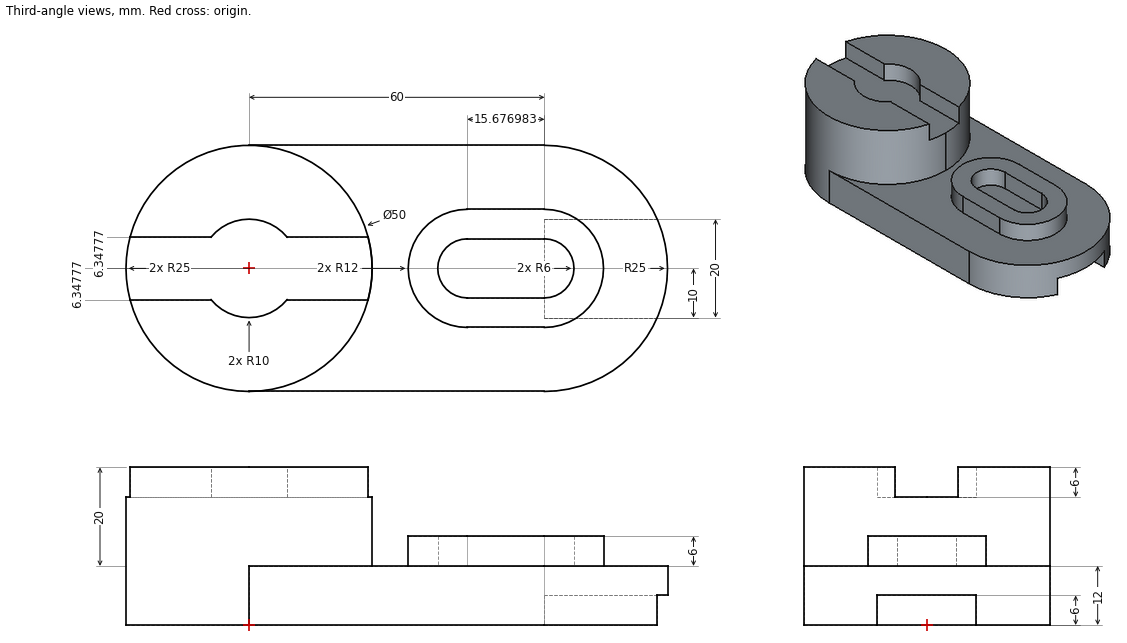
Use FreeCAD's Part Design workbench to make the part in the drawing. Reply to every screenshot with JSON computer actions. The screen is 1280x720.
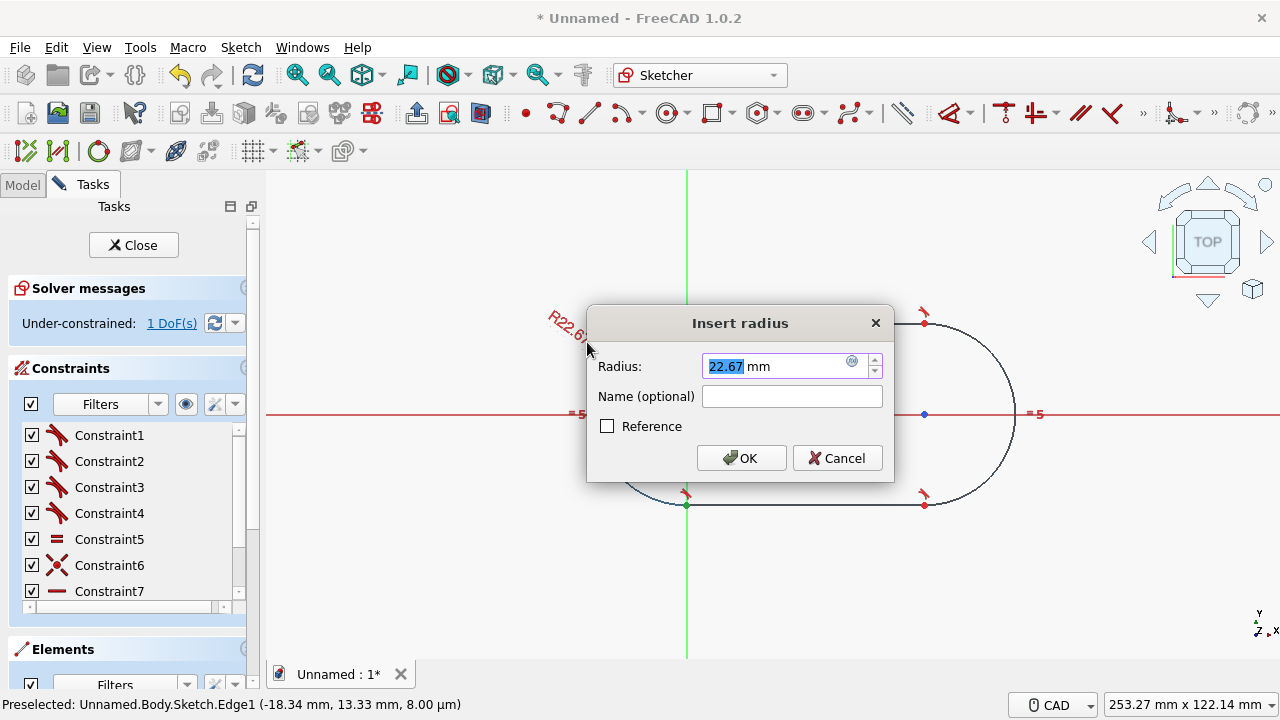
{"action": "type", "text": "25"}
{"action": "key", "text": "Return"}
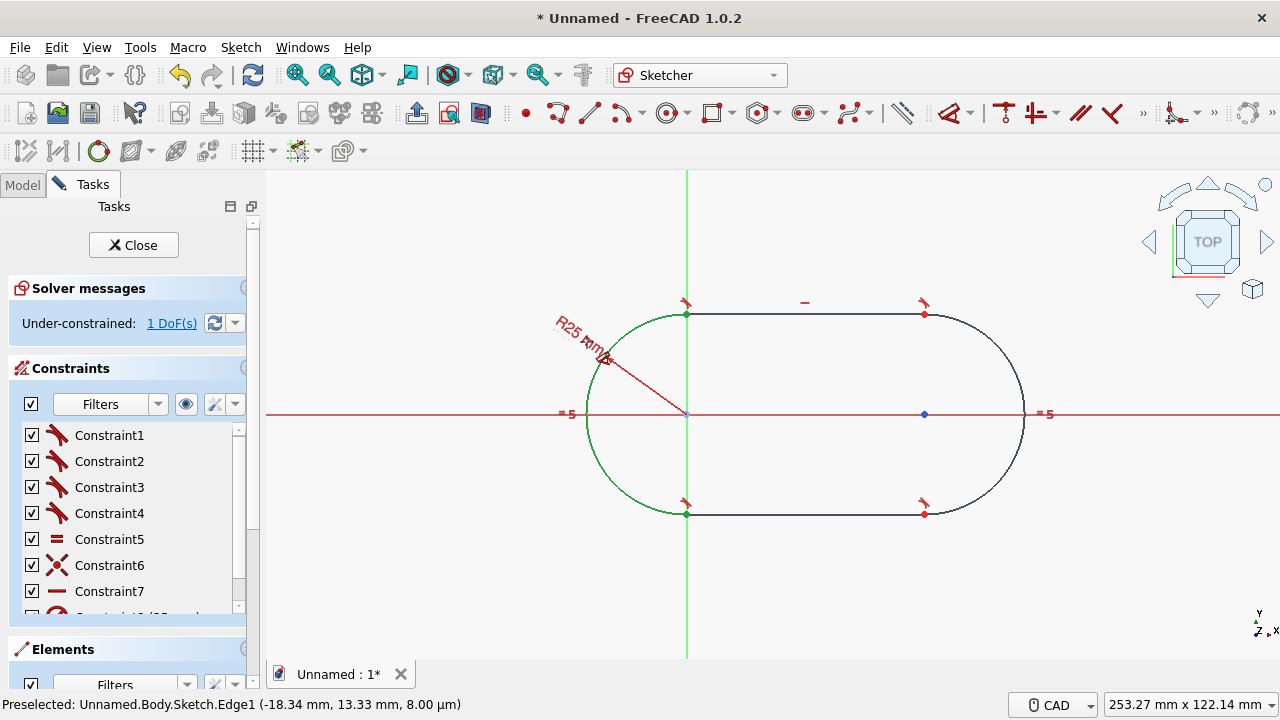
{"action": "left_click", "coordinate": [758, 314]}
{"action": "left_click", "coordinate": [806, 280]}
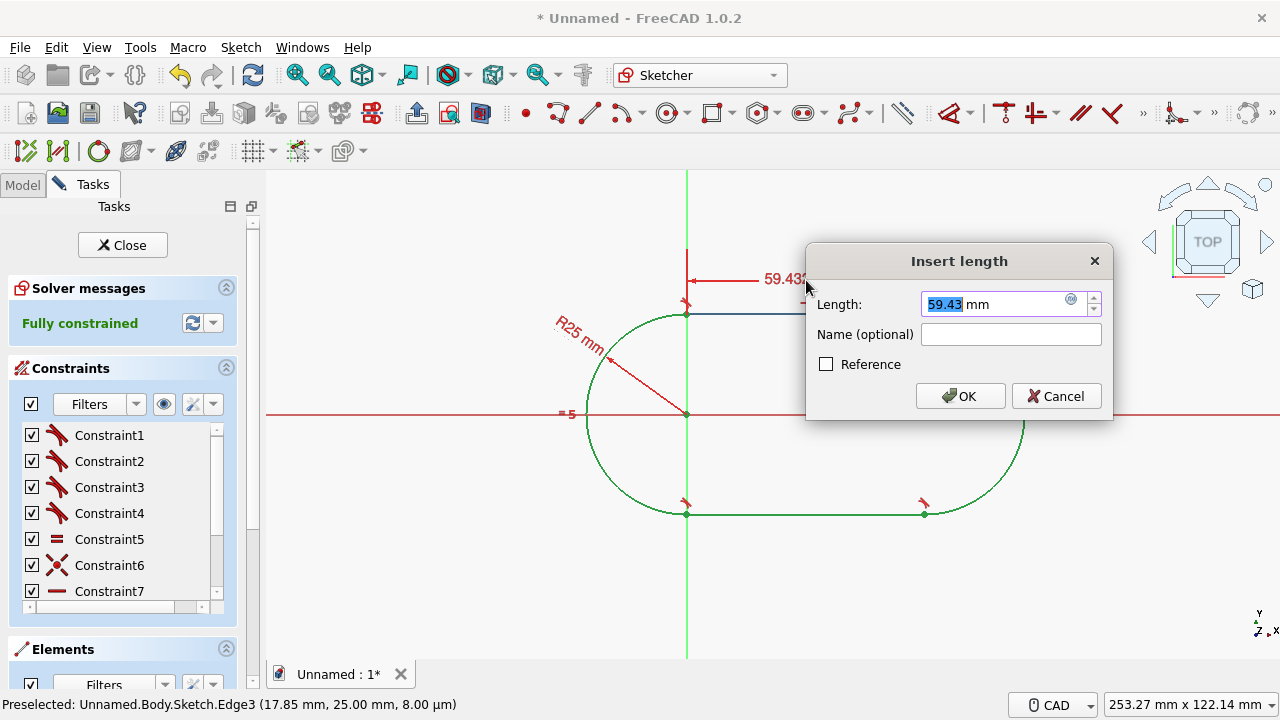
{"action": "type", "text": "60"}
{"action": "key", "text": "Return"}
{"action": "key", "text": "Escape"}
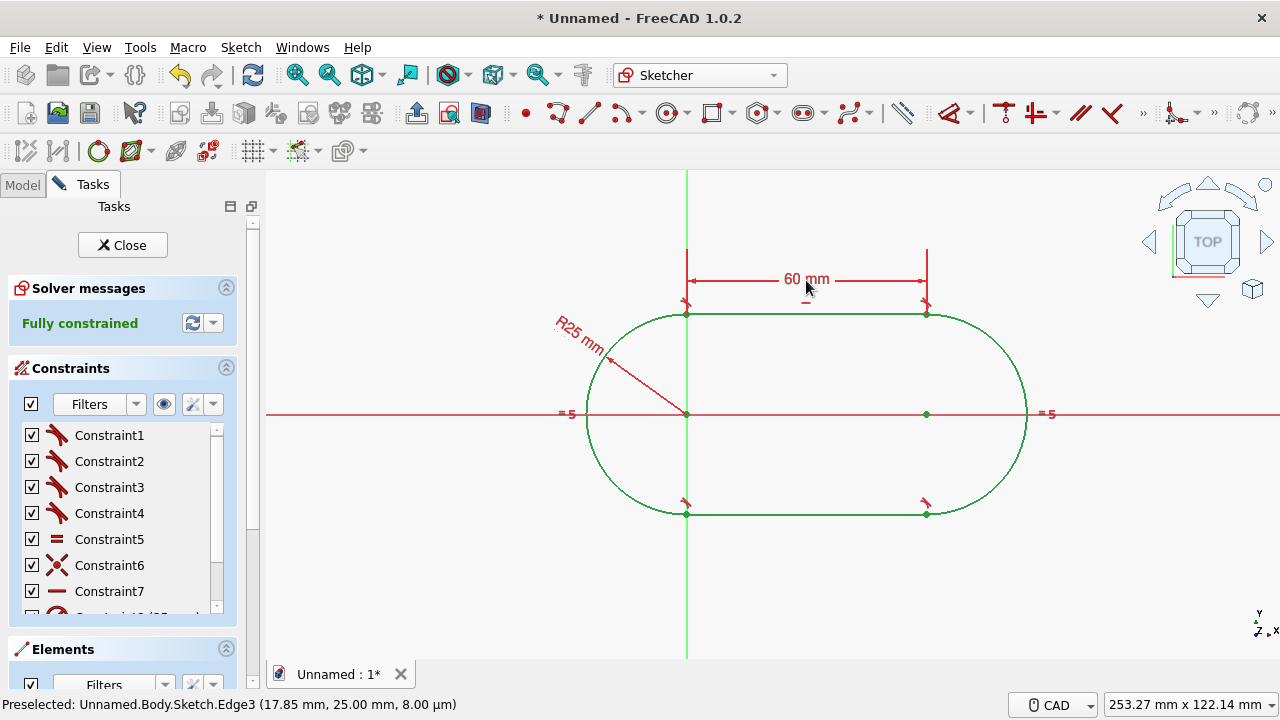
{"action": "left_click", "coordinate": [123, 245]}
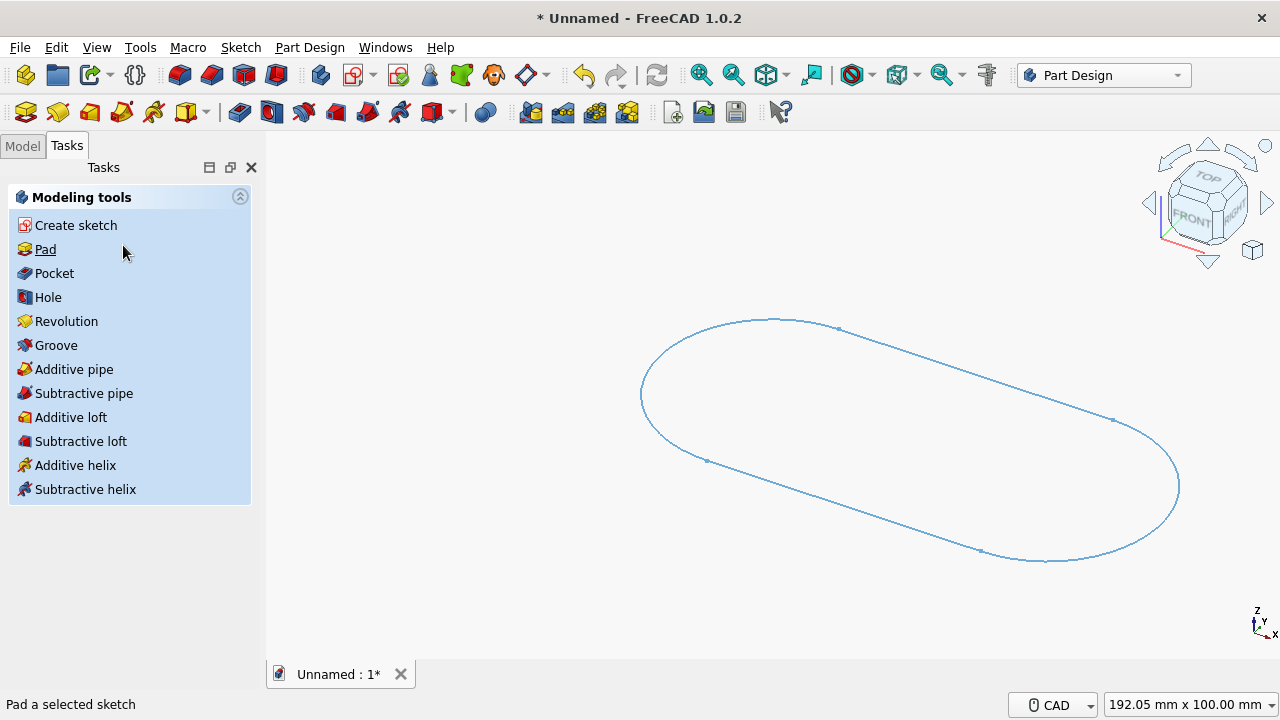
{"action": "left_click", "coordinate": [26, 112]}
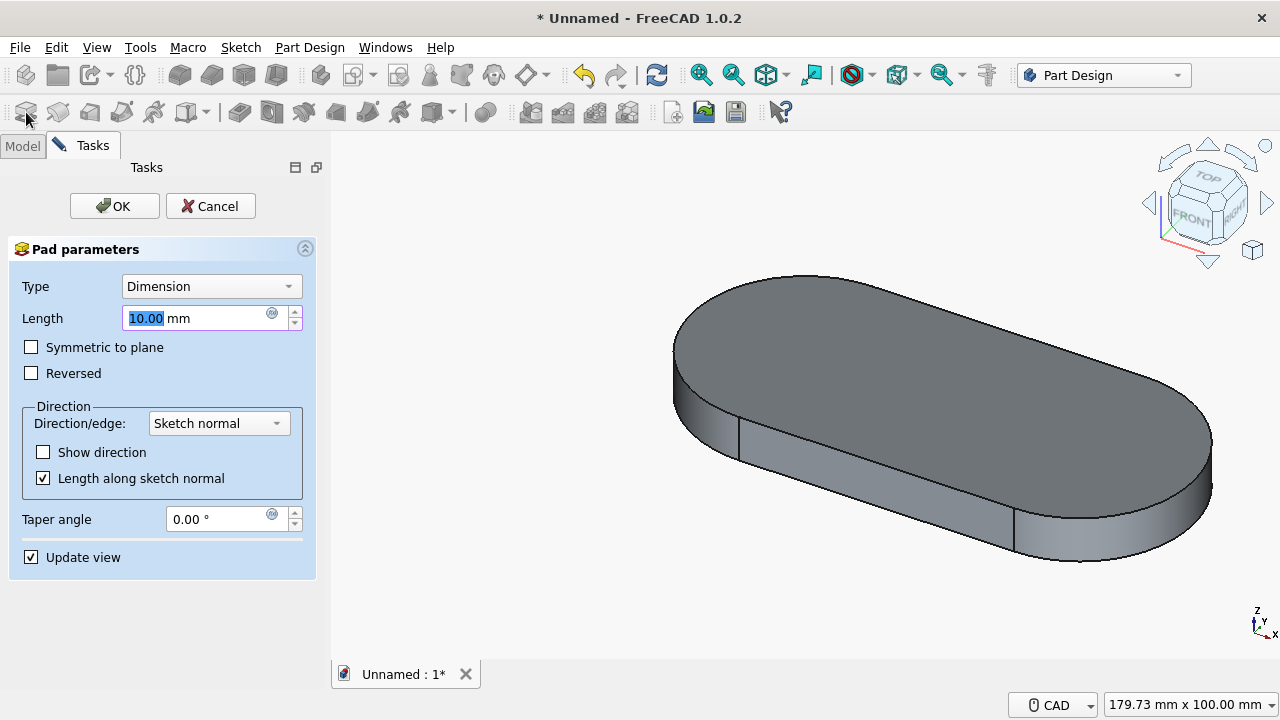
{"action": "type", "text": "12"}
{"action": "key", "text": "Tab"}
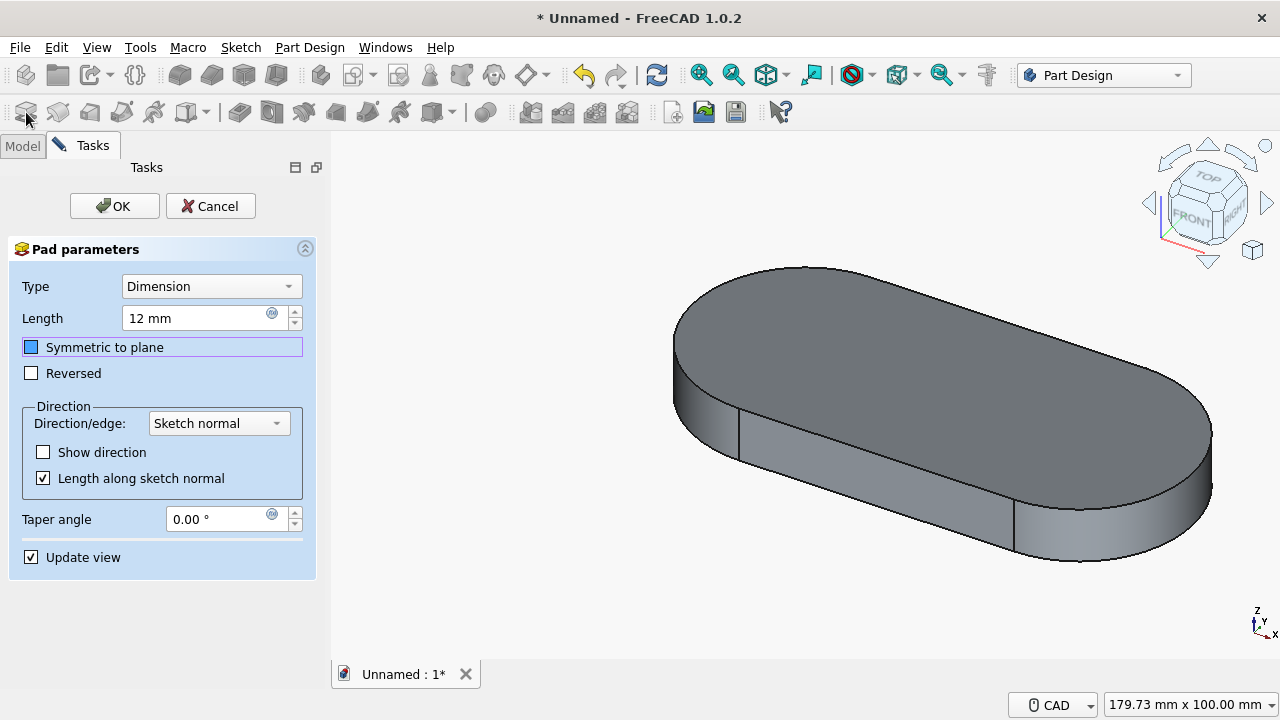
{"action": "left_click", "coordinate": [115, 206]}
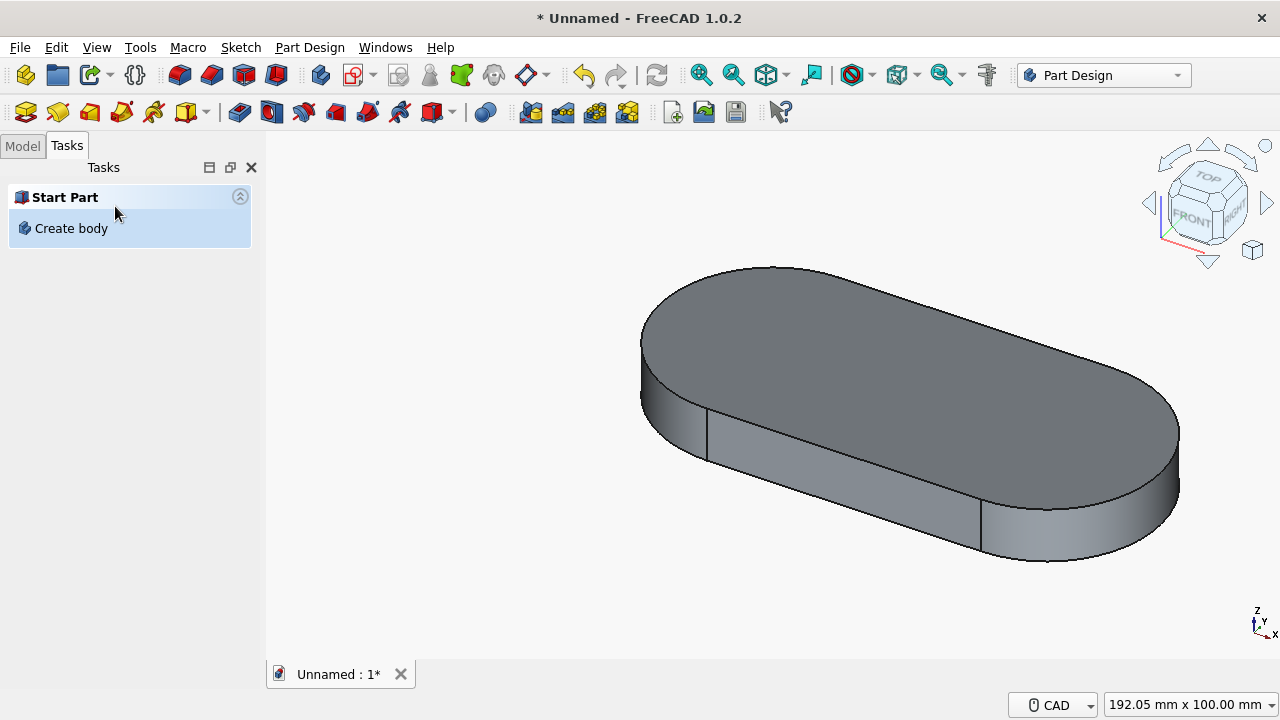
{"action": "left_click", "coordinate": [982, 411]}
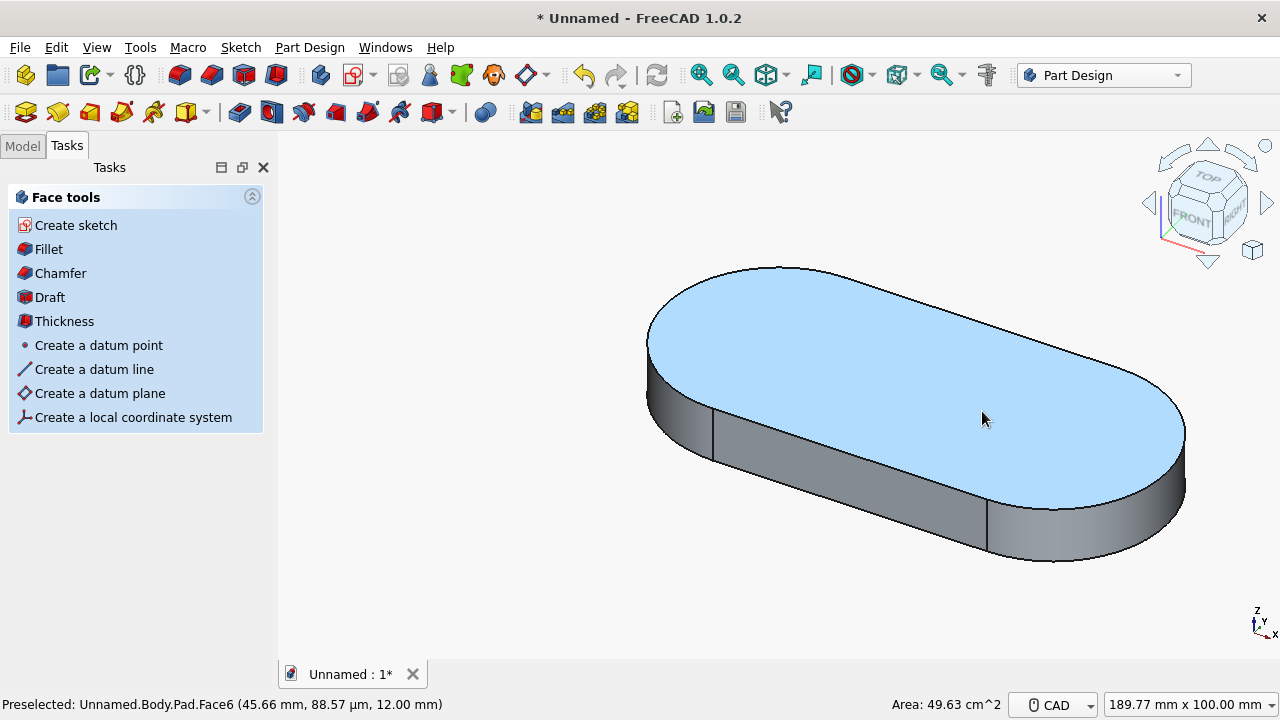
{"action": "left_click", "coordinate": [354, 76]}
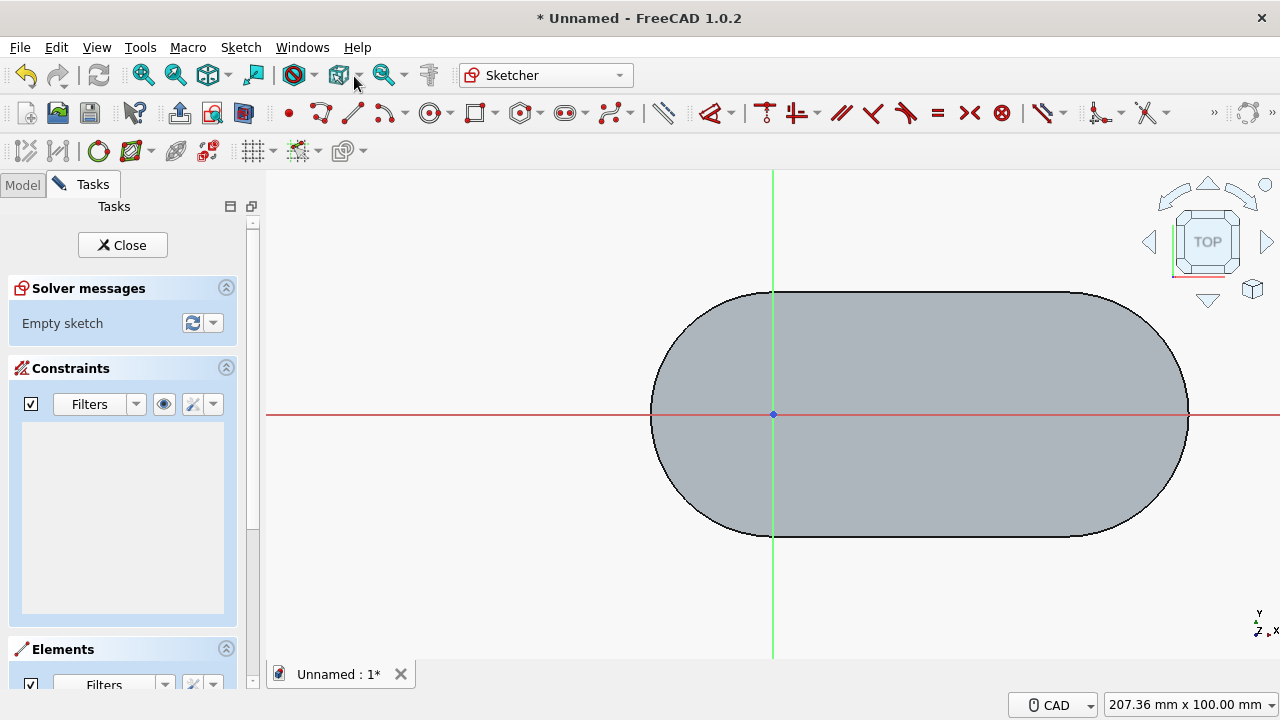
{"action": "key", "text": "g c"}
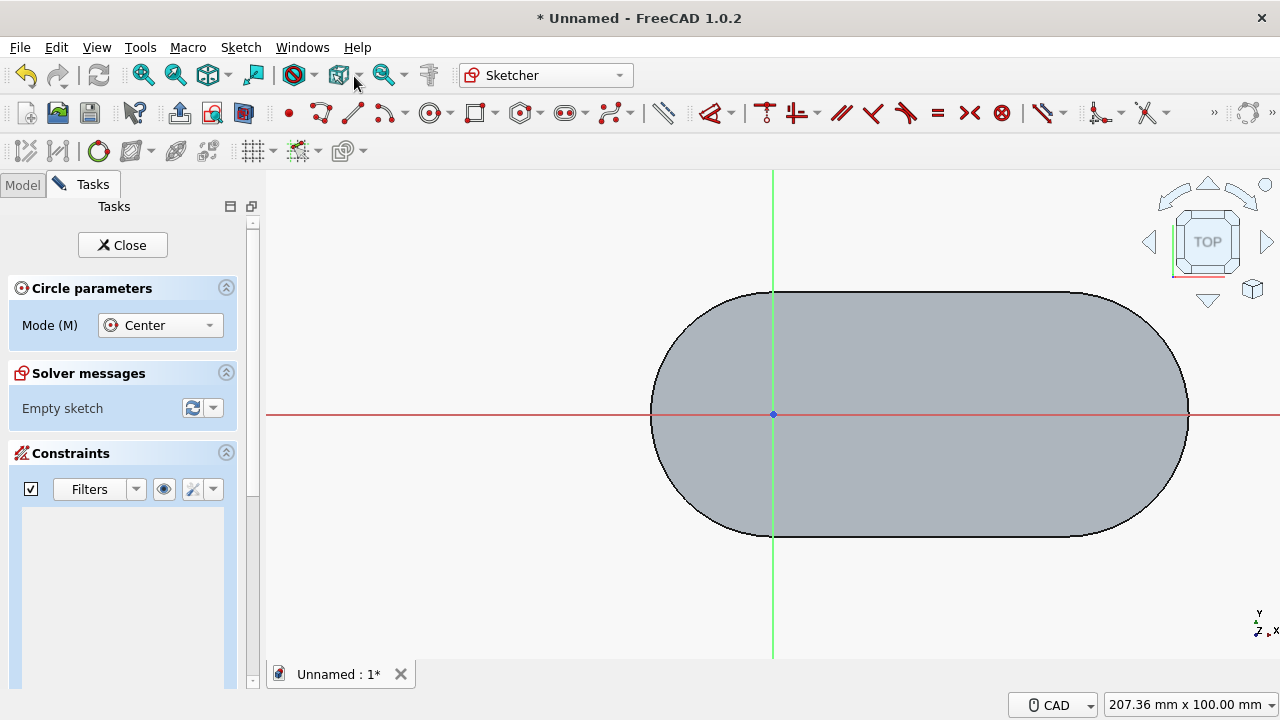
{"action": "left_click", "coordinate": [773, 414]}
{"action": "left_click", "coordinate": [859, 328]}
{"action": "key", "text": "Escape"}